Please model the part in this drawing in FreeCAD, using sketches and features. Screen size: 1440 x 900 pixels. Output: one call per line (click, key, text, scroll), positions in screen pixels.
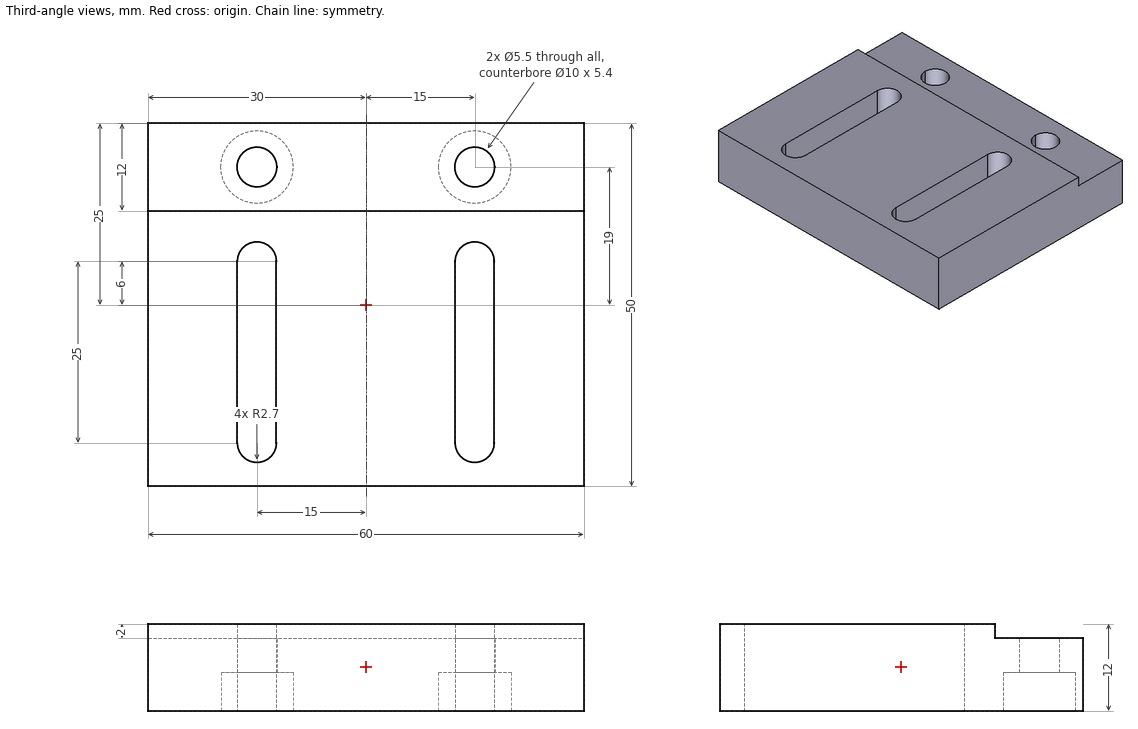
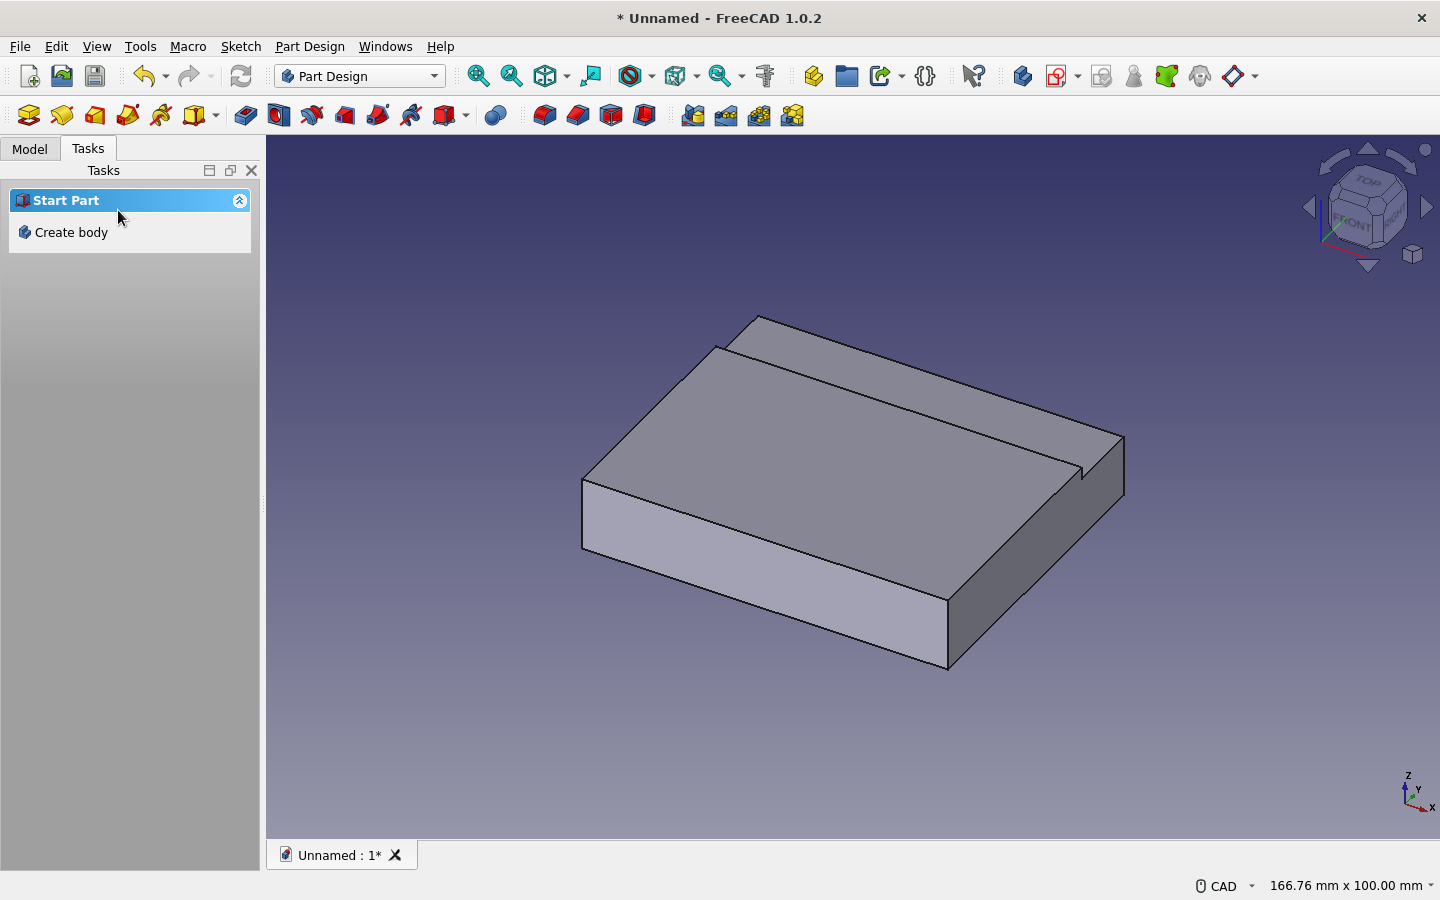
click(884, 490)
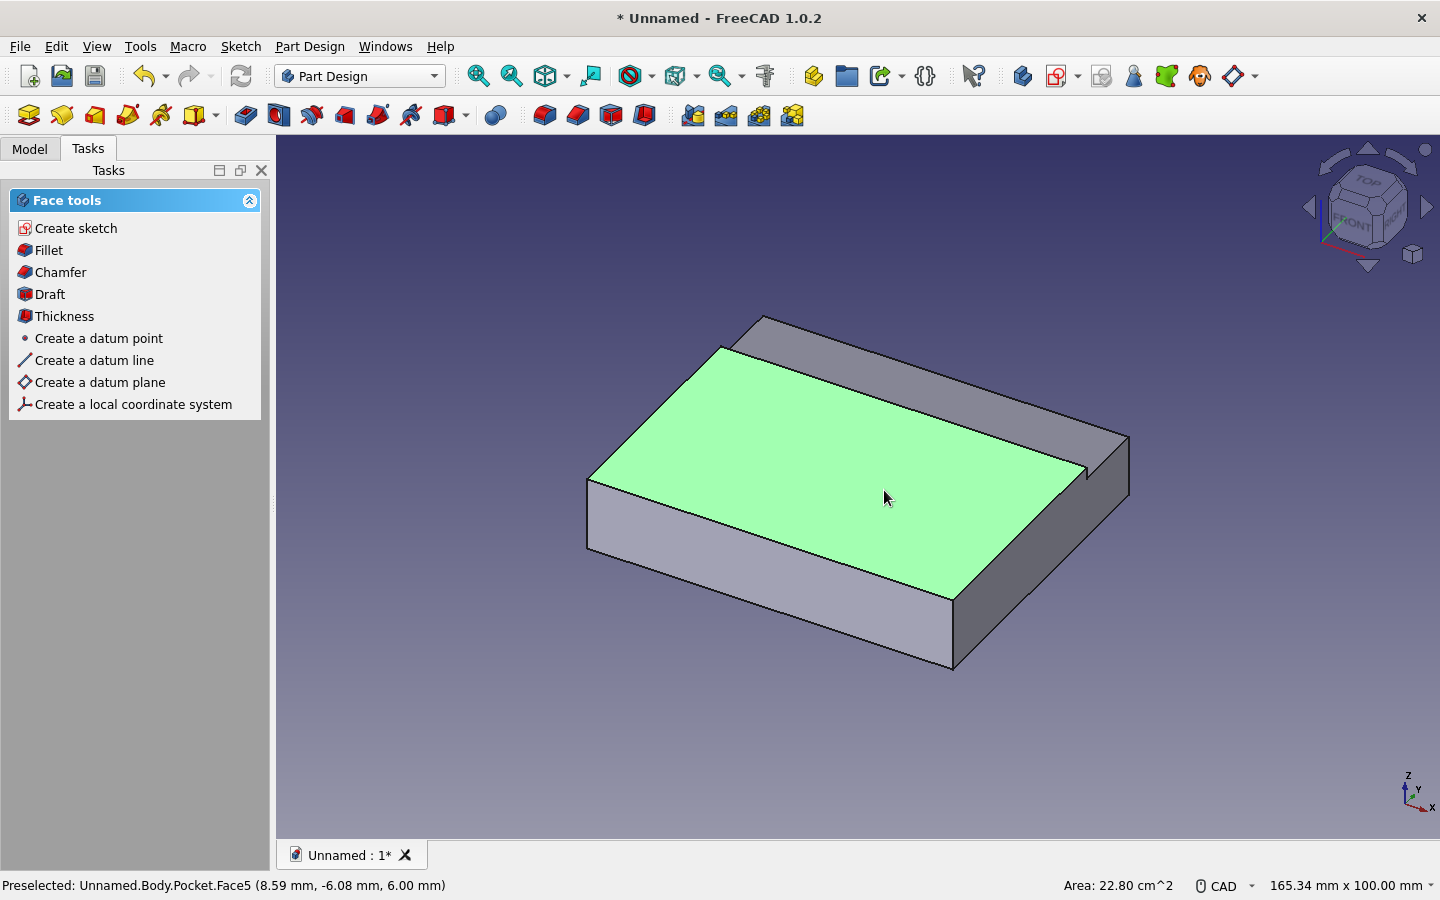
click(1056, 76)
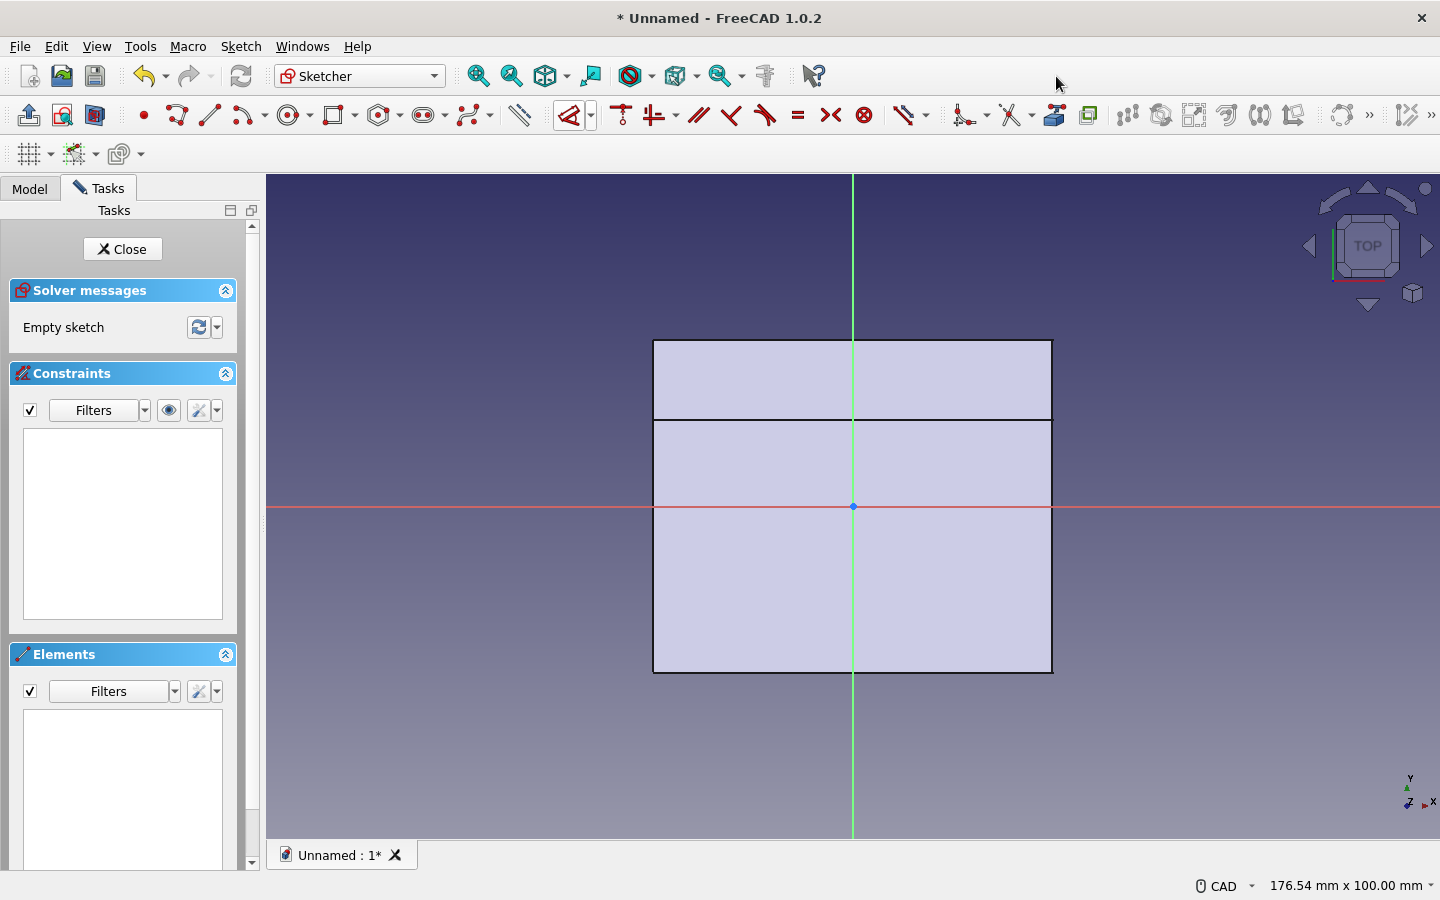
scroll(909, 585, up, 4)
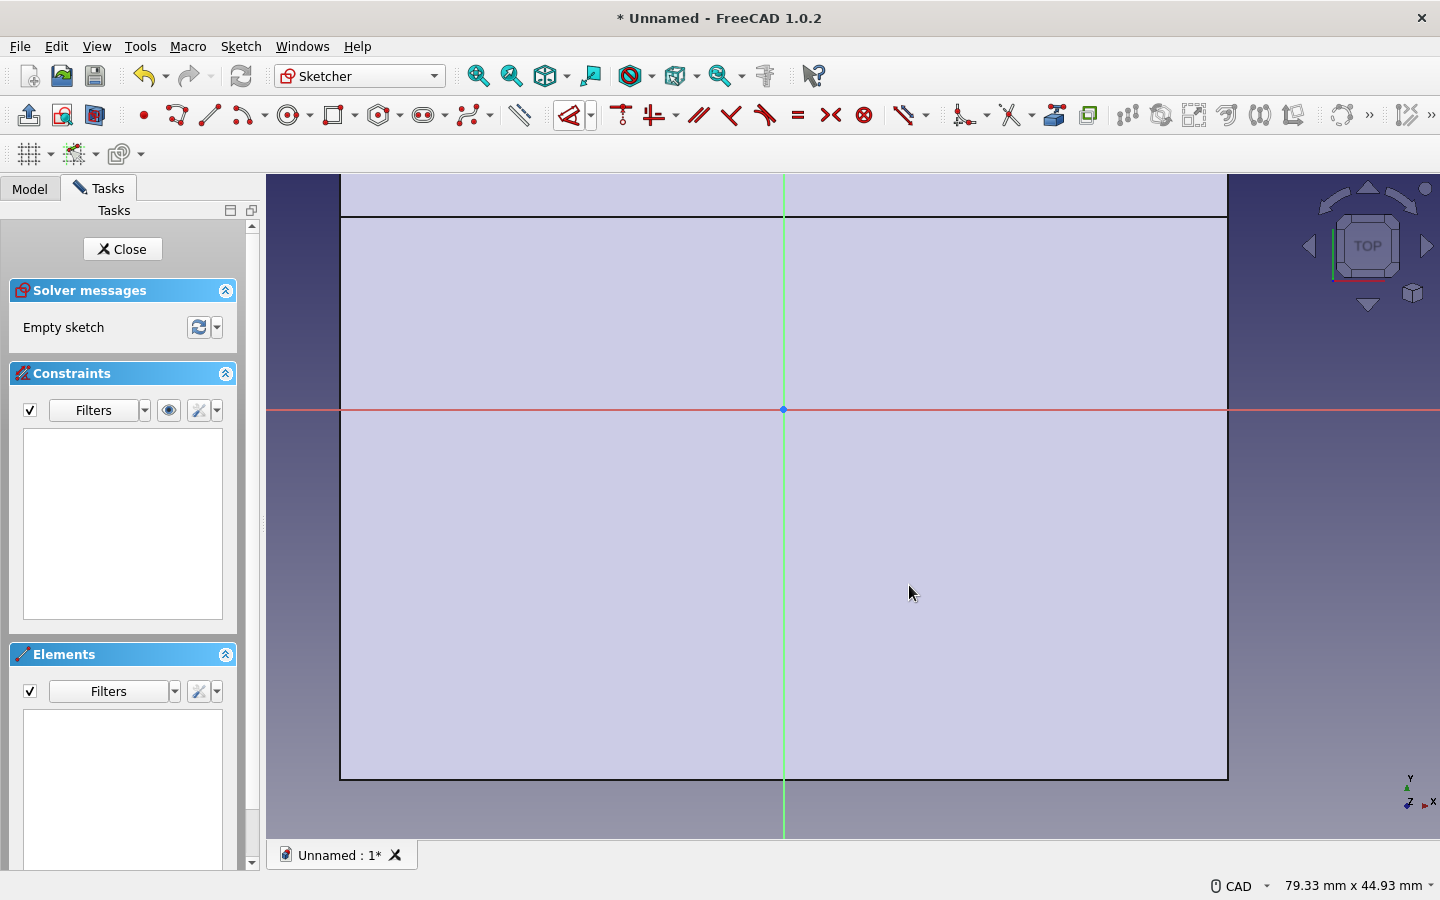
click(422, 116)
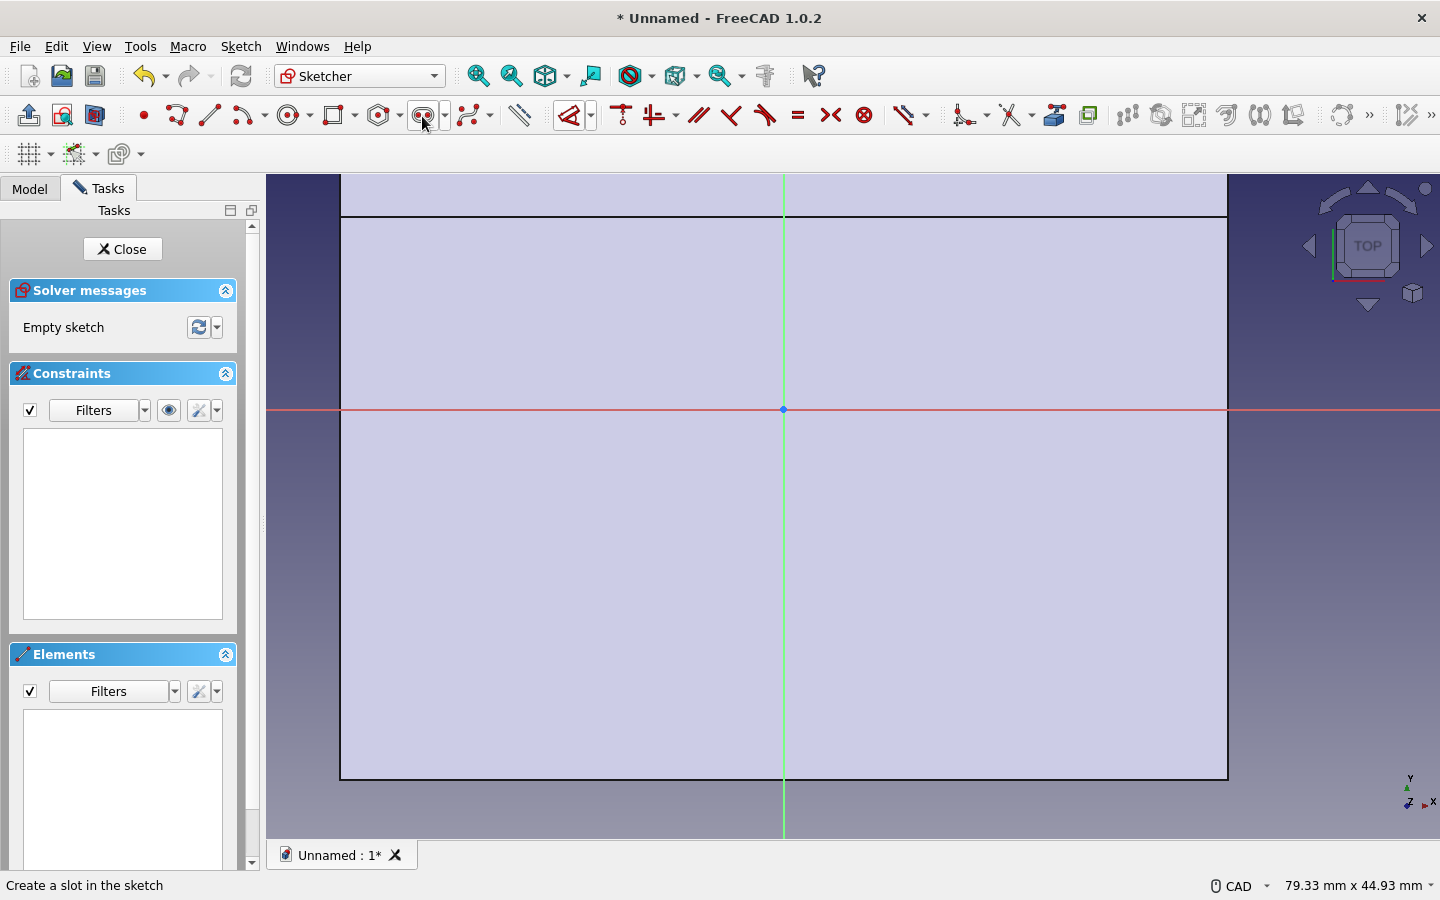
click(562, 691)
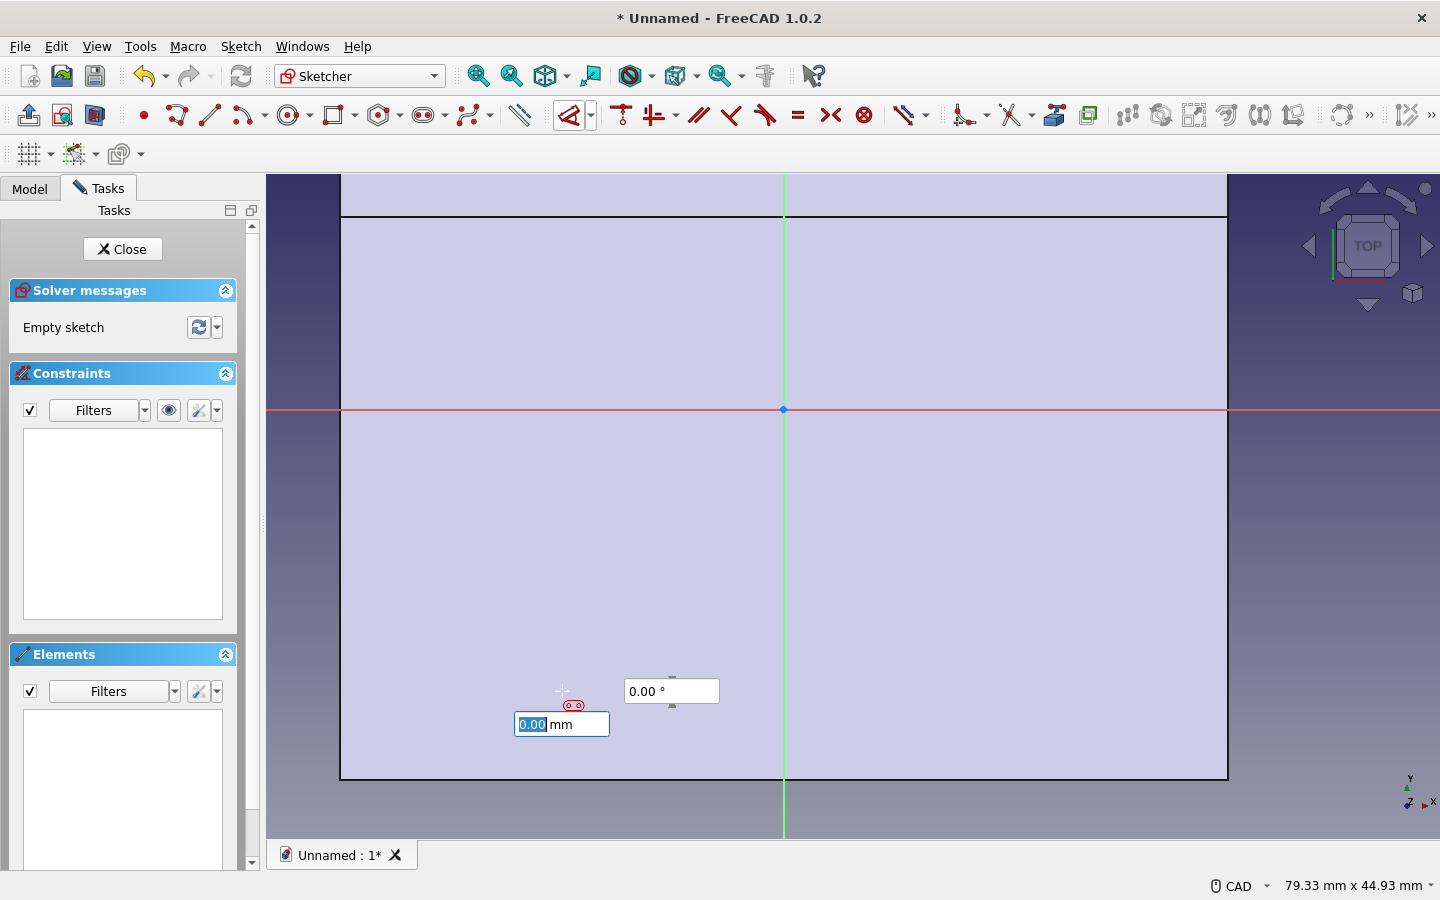
click(562, 321)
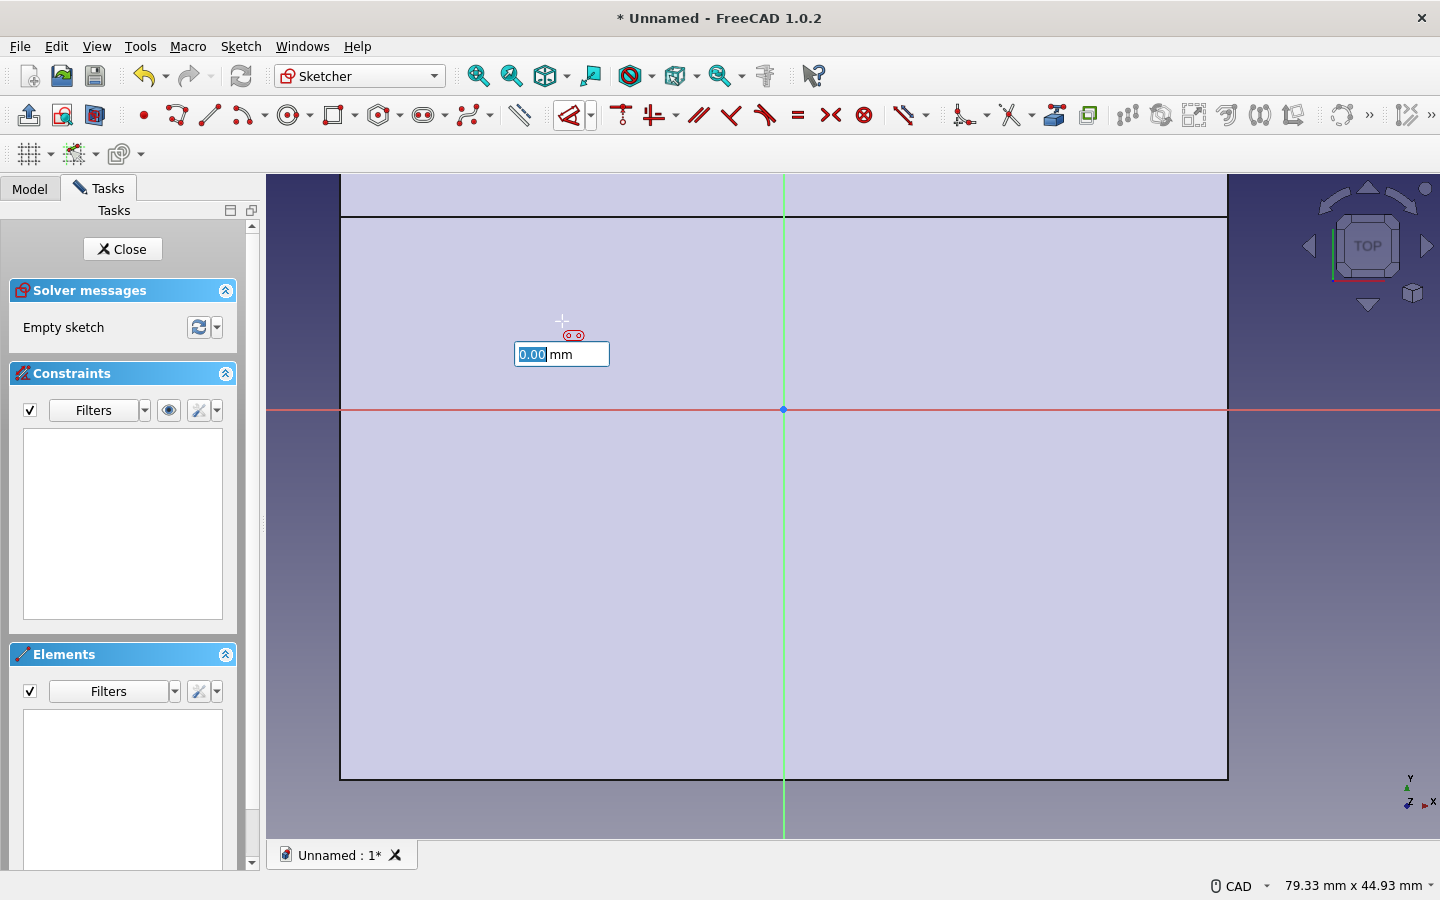
click(522, 506)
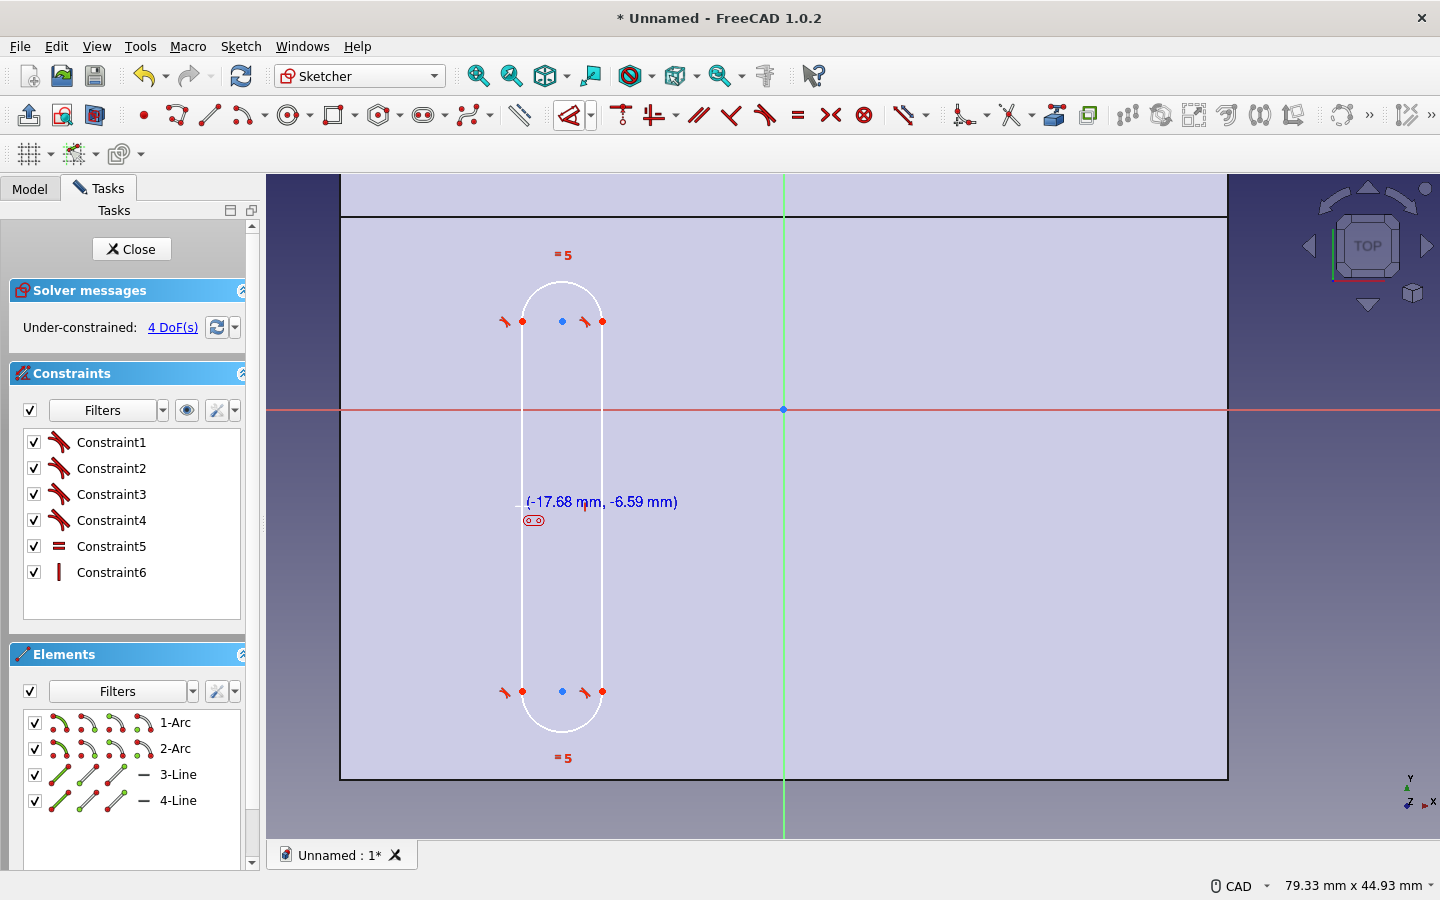
click(1006, 691)